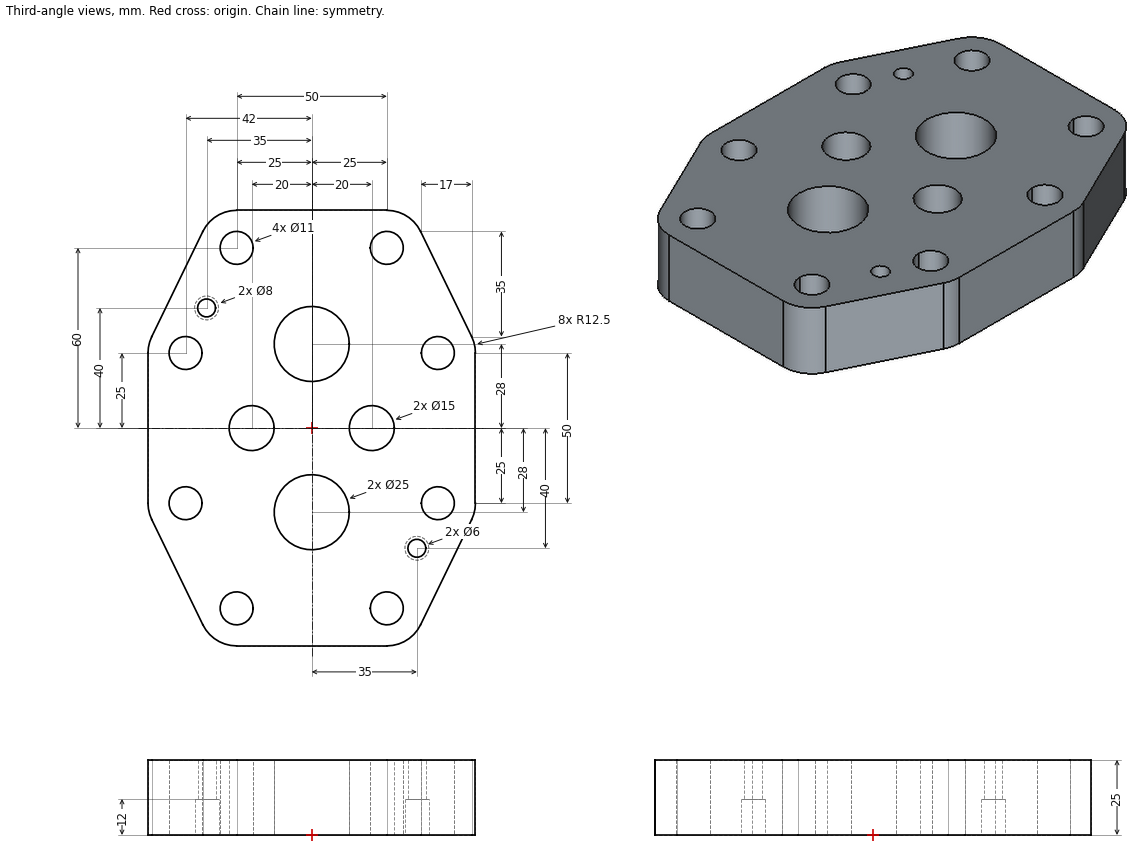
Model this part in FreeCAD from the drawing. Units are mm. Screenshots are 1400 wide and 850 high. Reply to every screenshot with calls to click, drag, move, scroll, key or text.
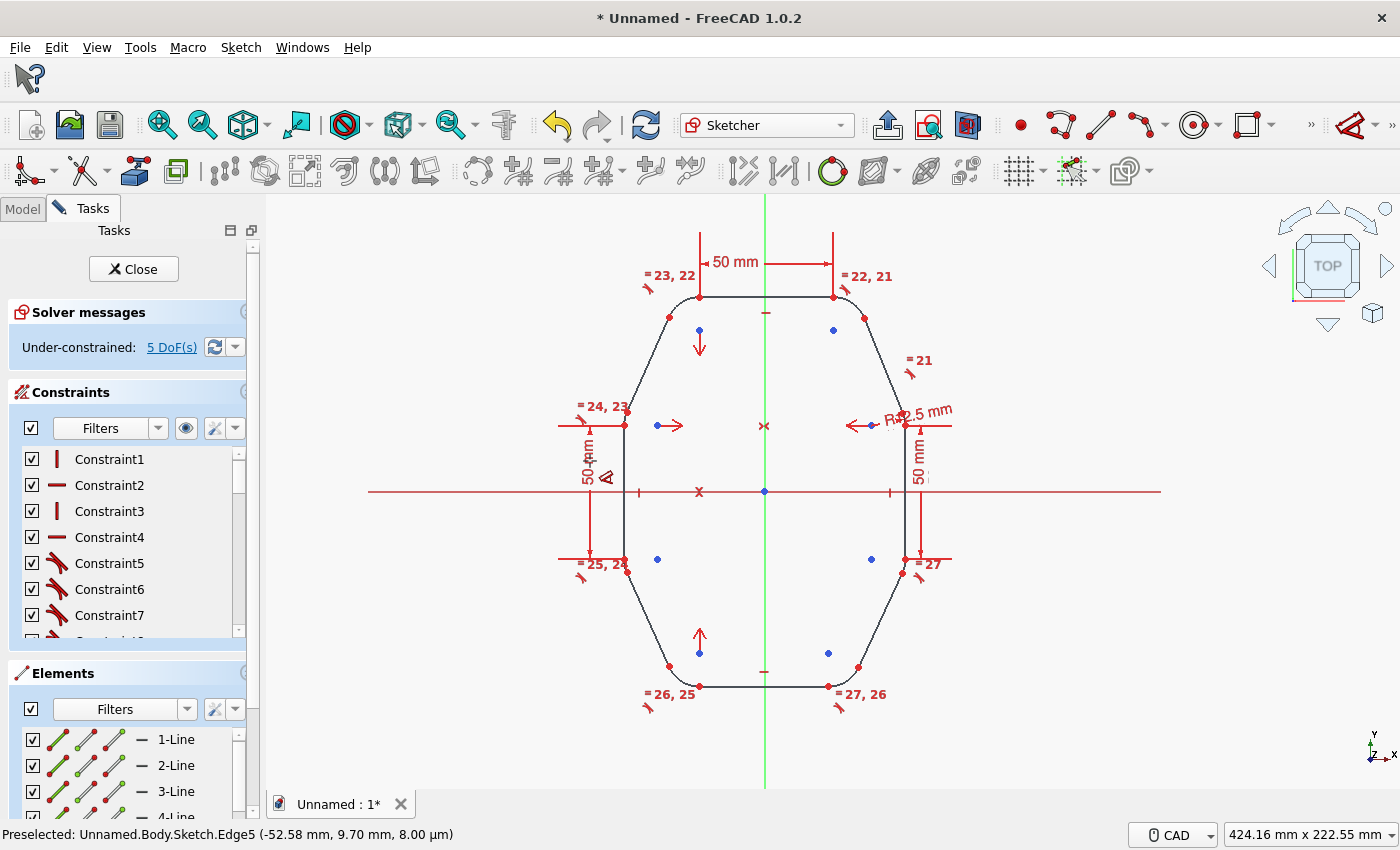
click(738, 687)
click(734, 721)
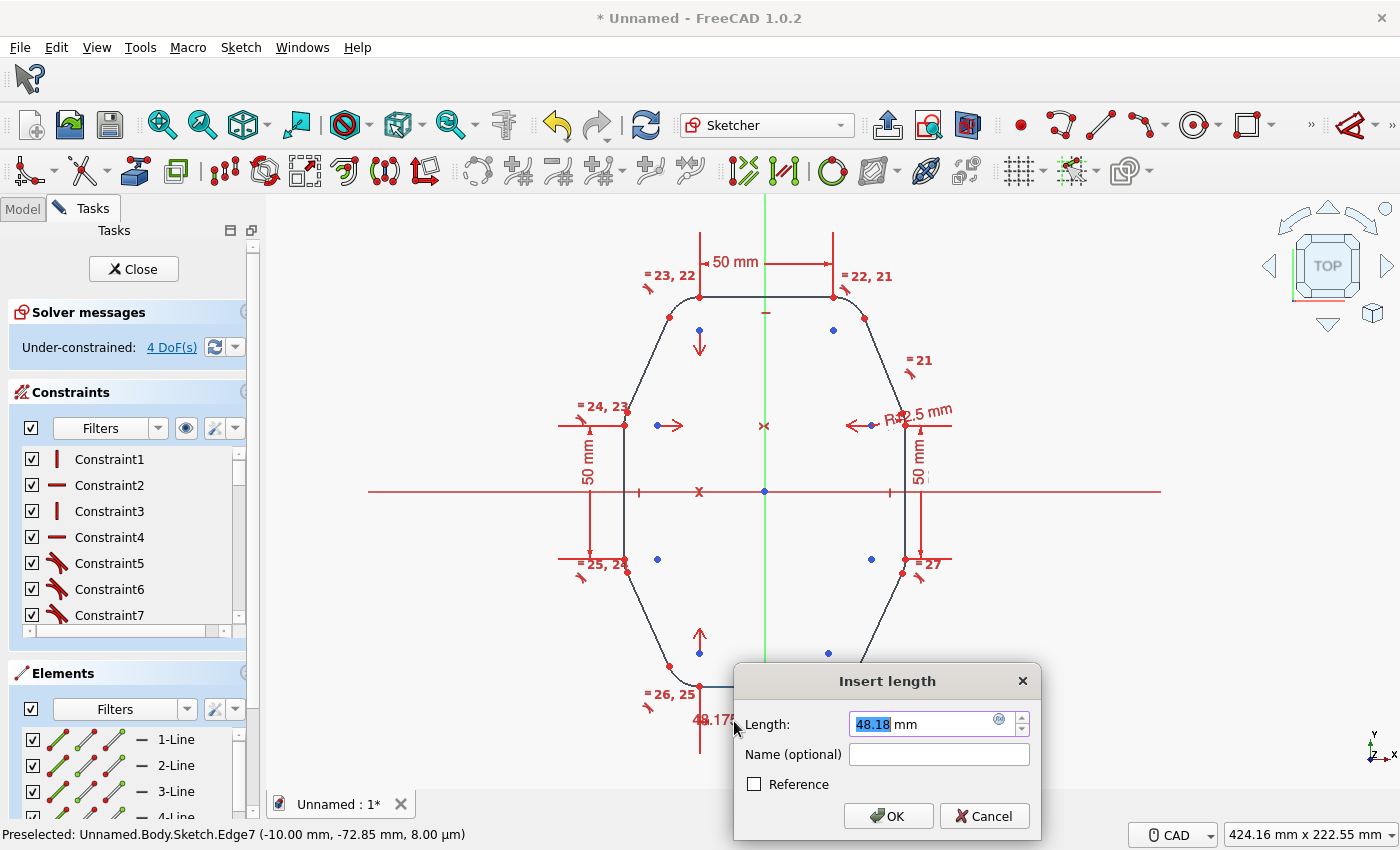
text(50)
key(Return)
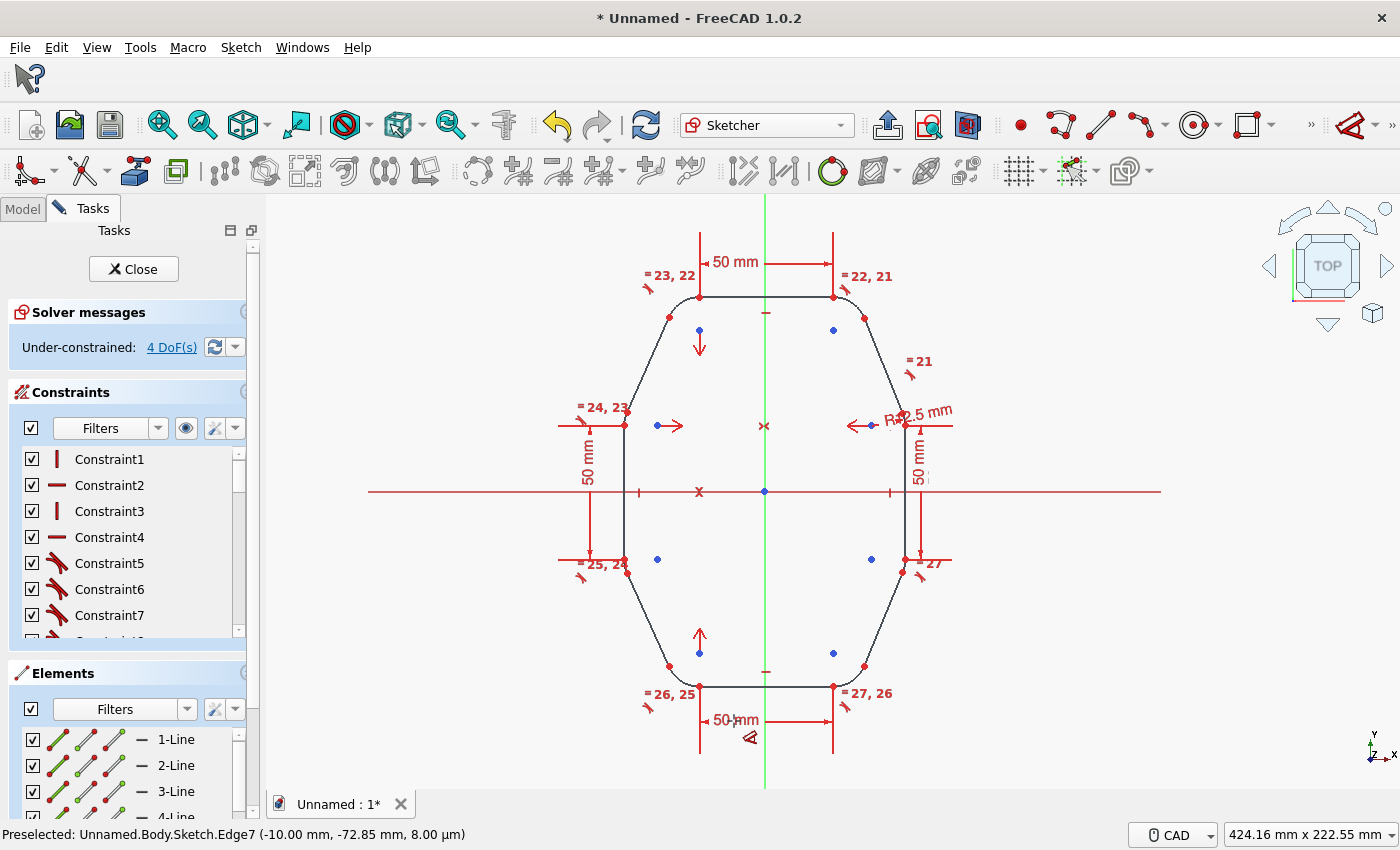
click(905, 560)
click(939, 526)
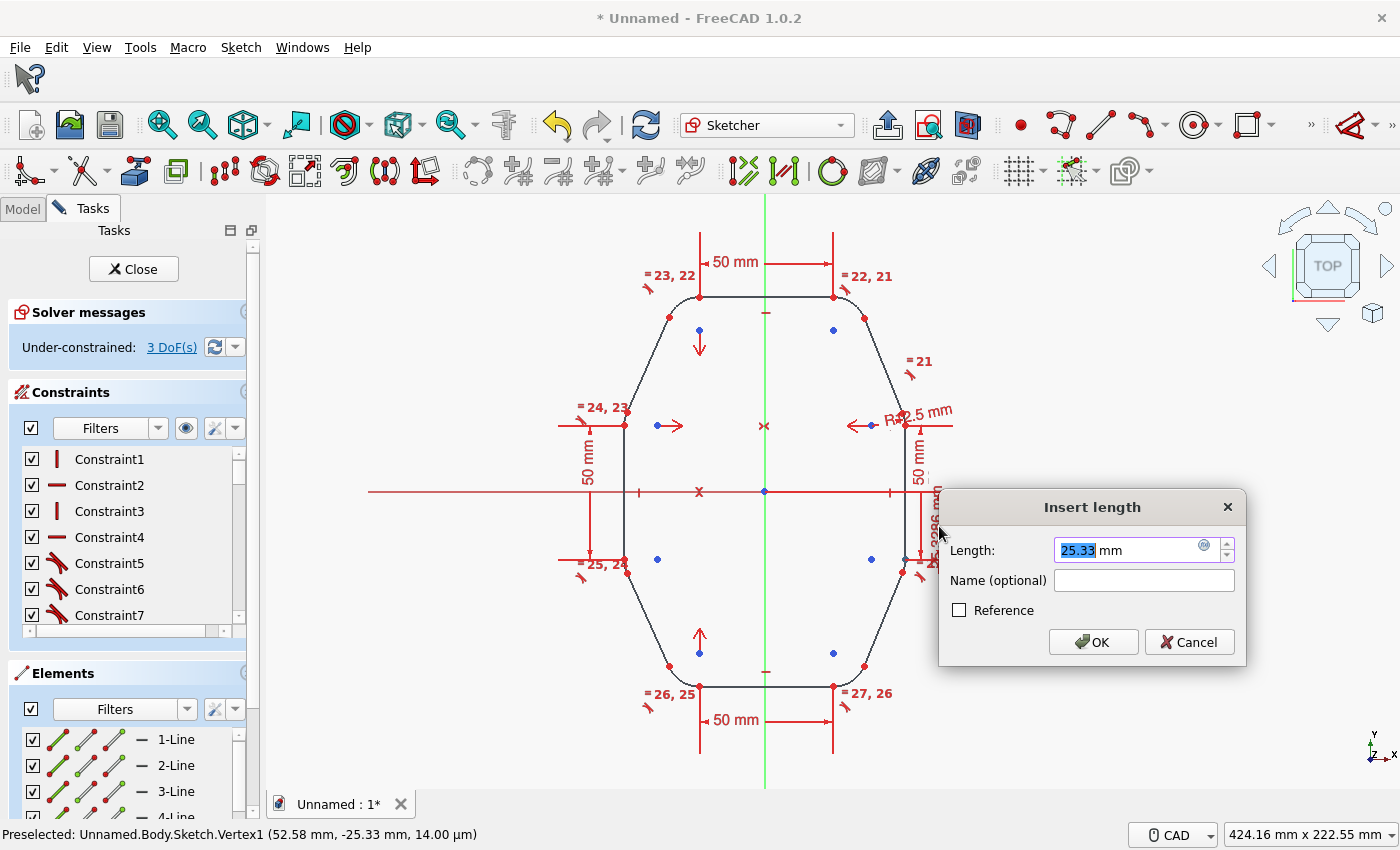
text(25)
key(Return)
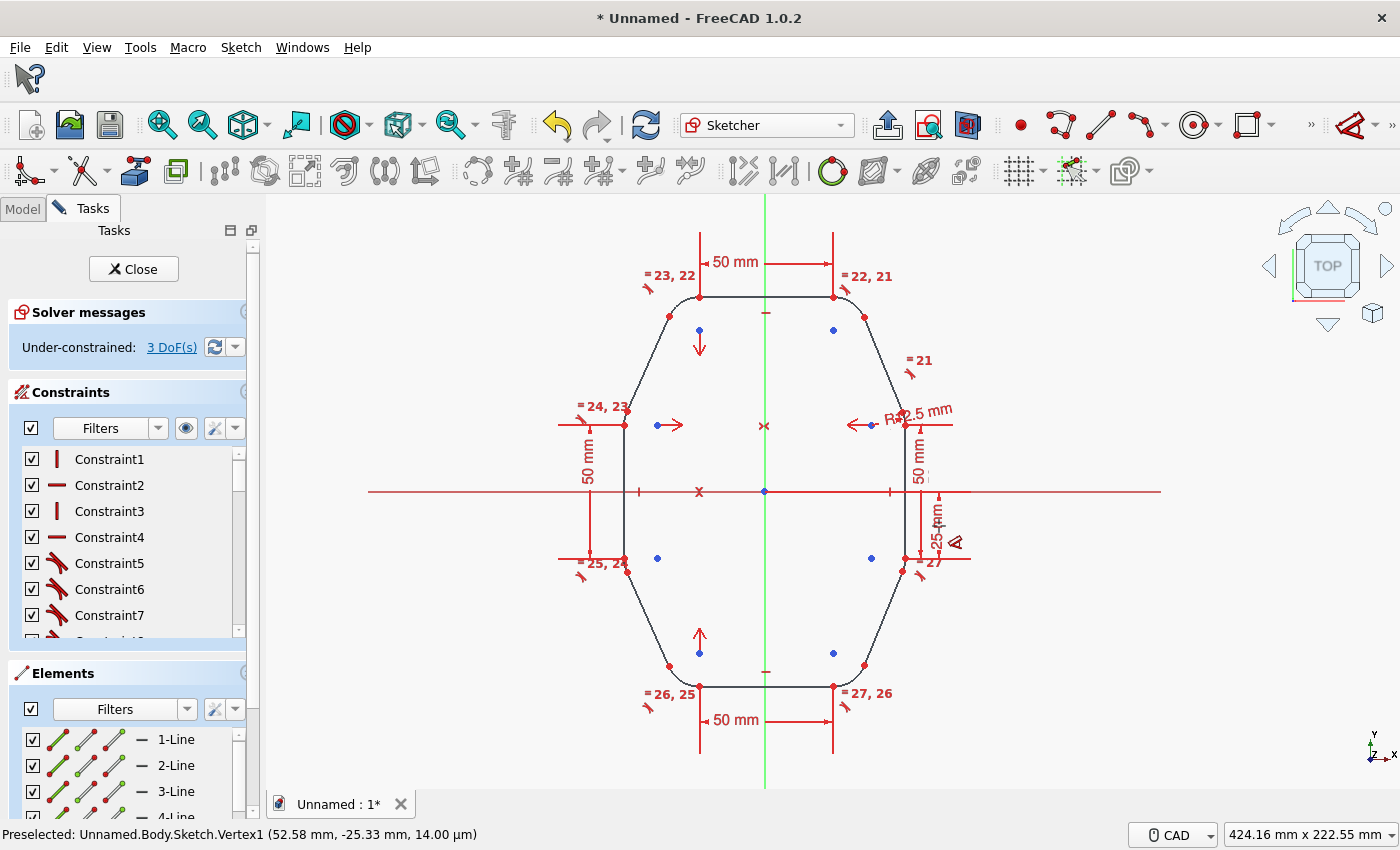
click(833, 297)
click(815, 263)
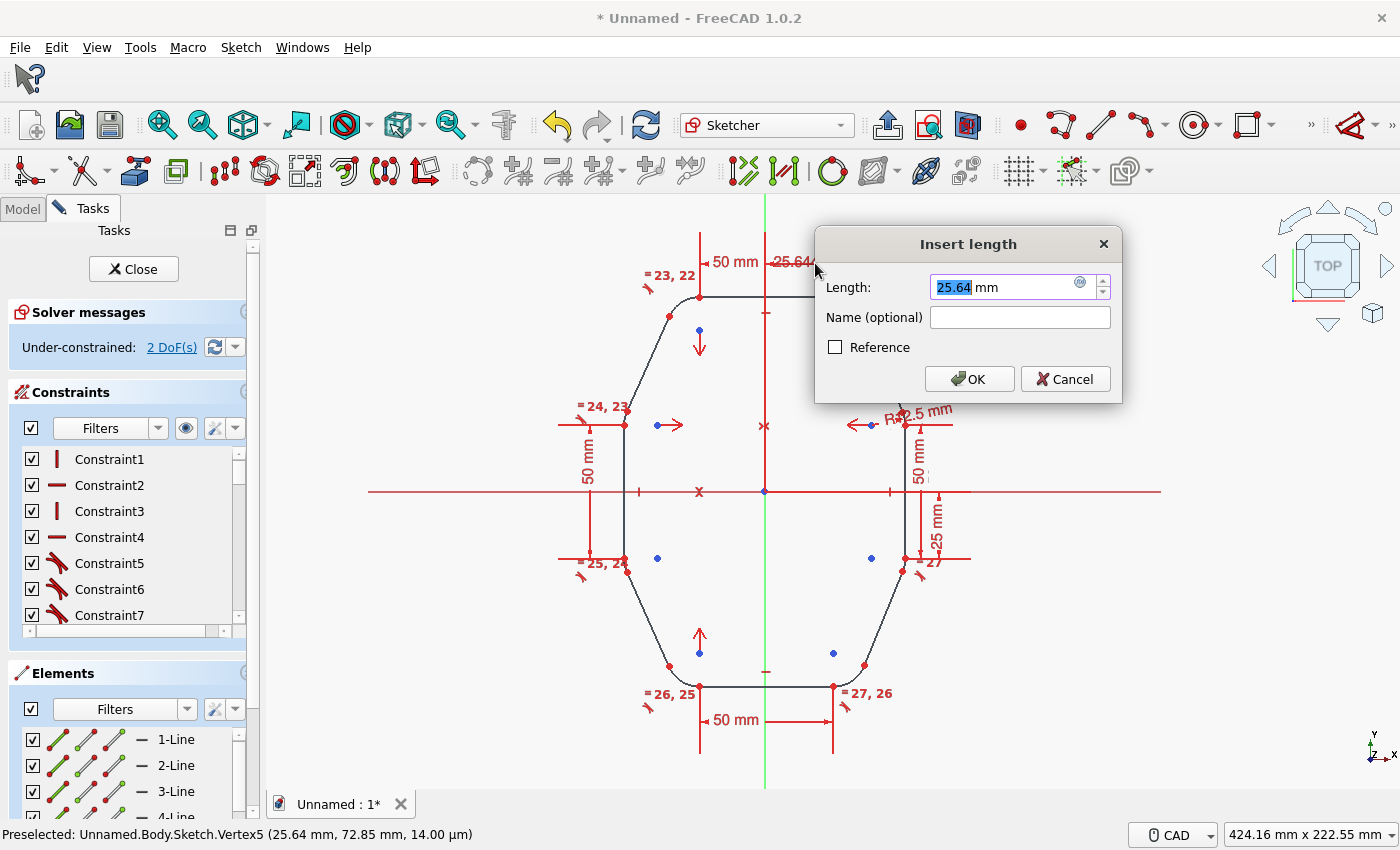
text(25)
key(Return)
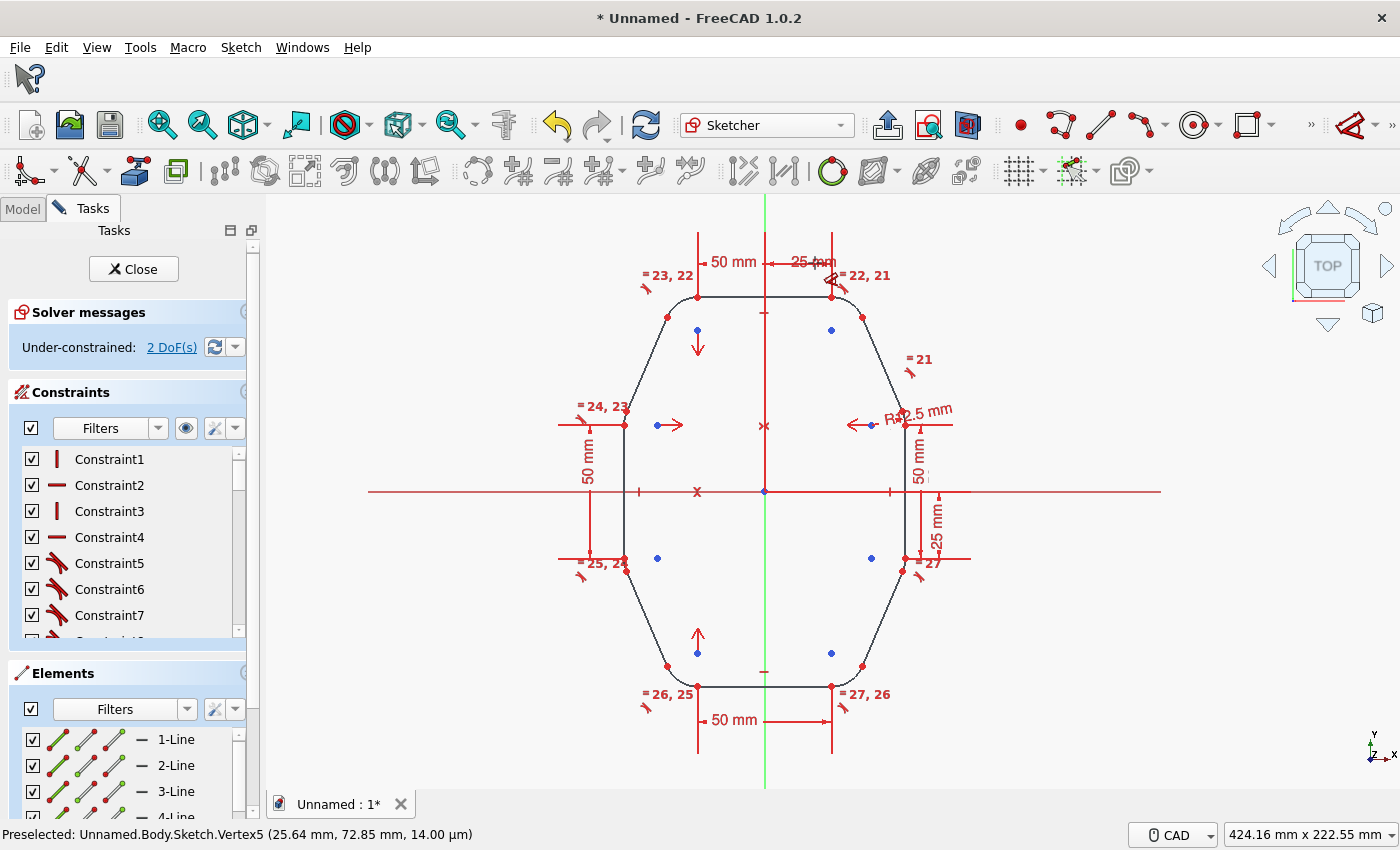
click(891, 384)
click(882, 283)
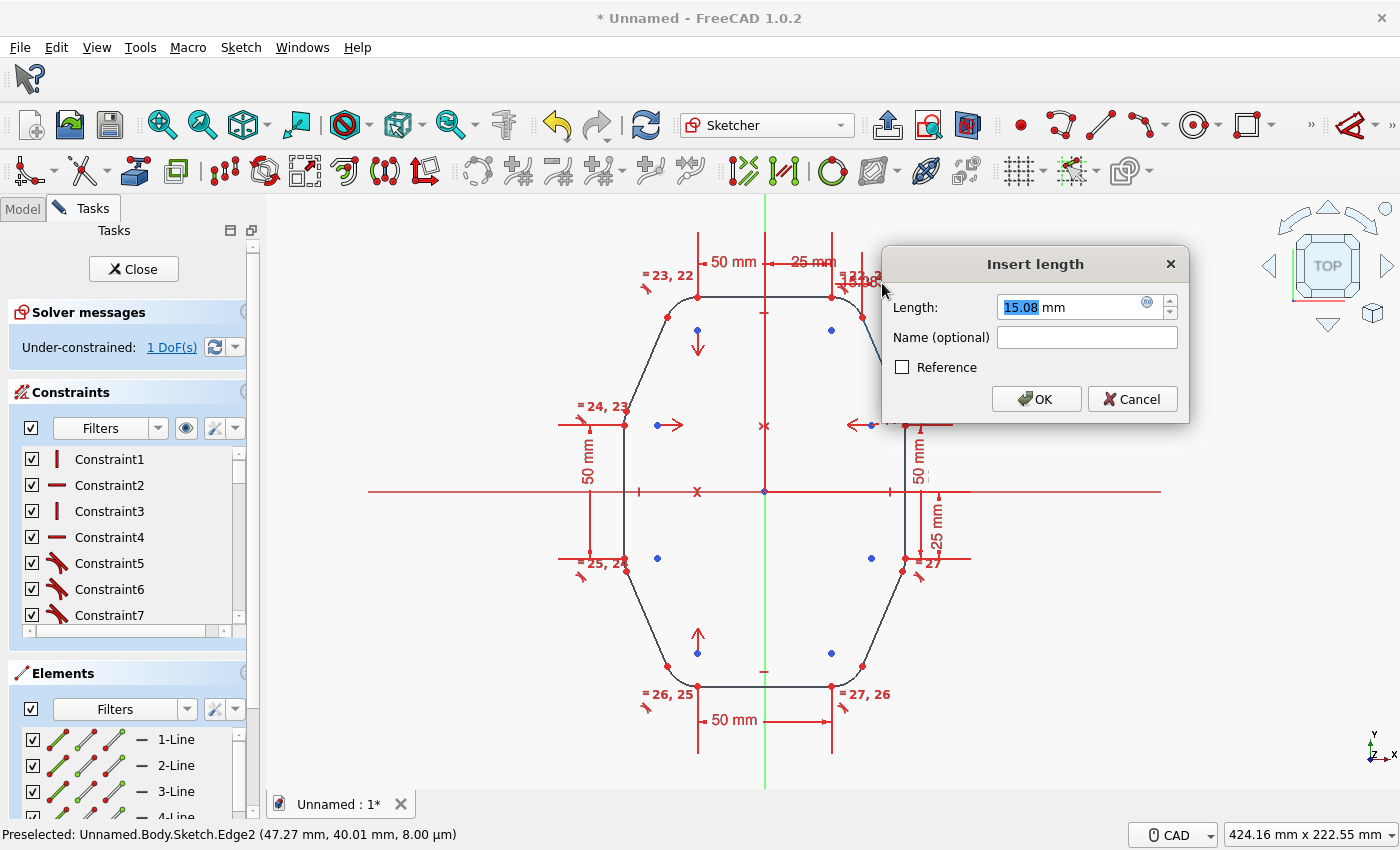
text(17)
key(Return)